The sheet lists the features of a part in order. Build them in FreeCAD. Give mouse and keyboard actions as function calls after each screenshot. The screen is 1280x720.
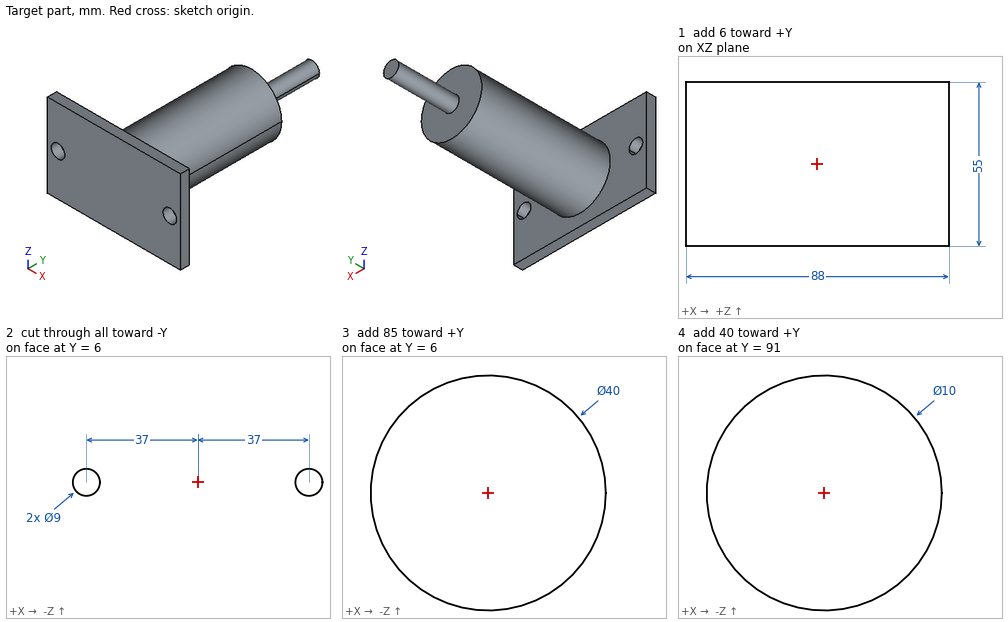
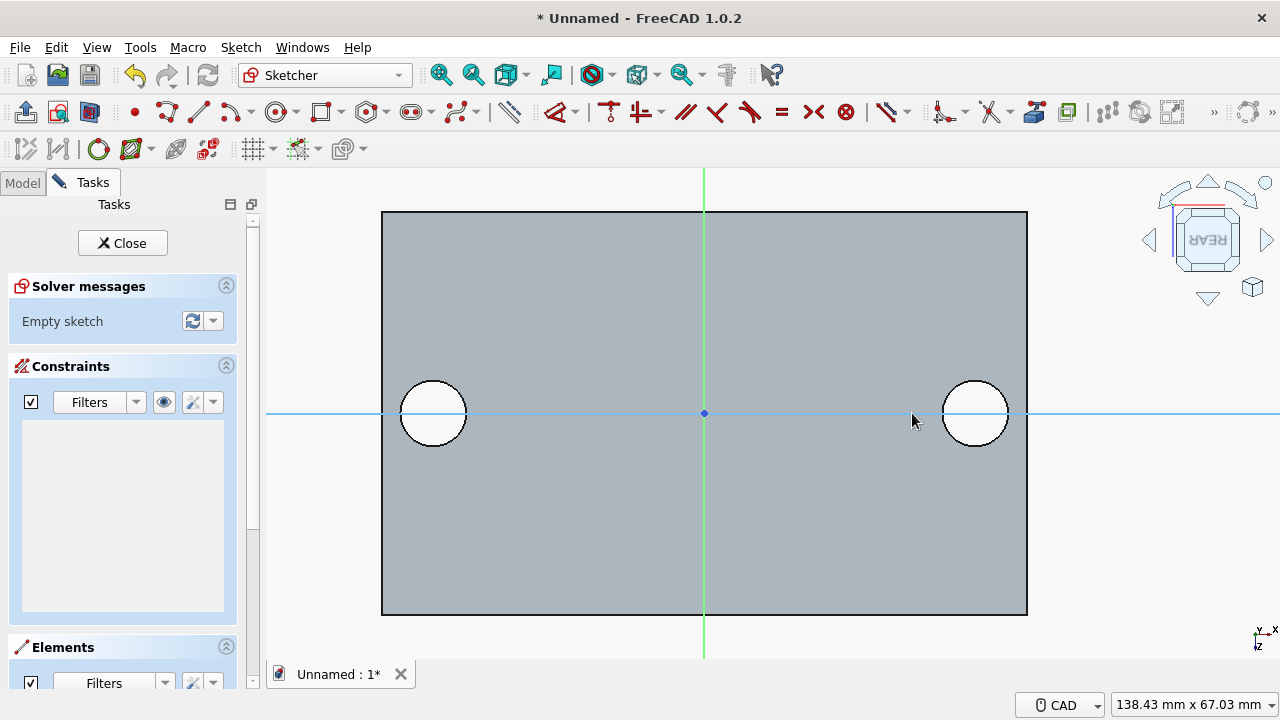
key(g)
key(c)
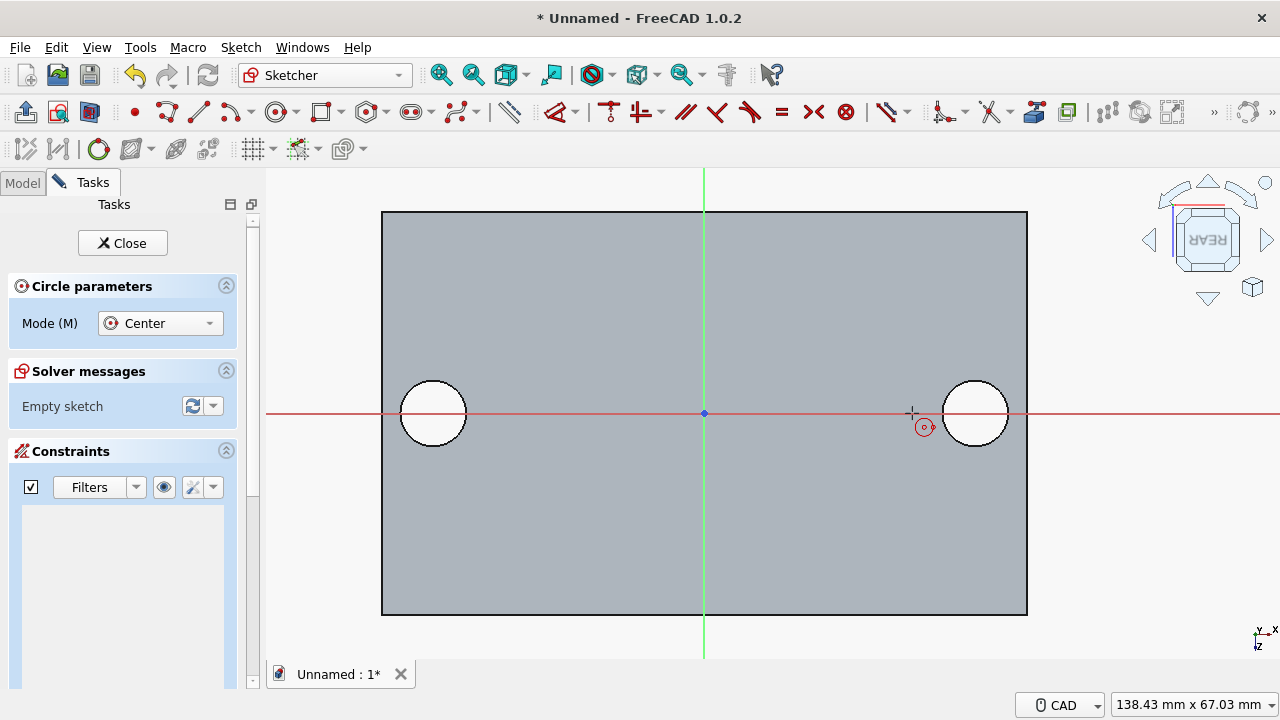
click(704, 413)
click(808, 310)
key(Escape)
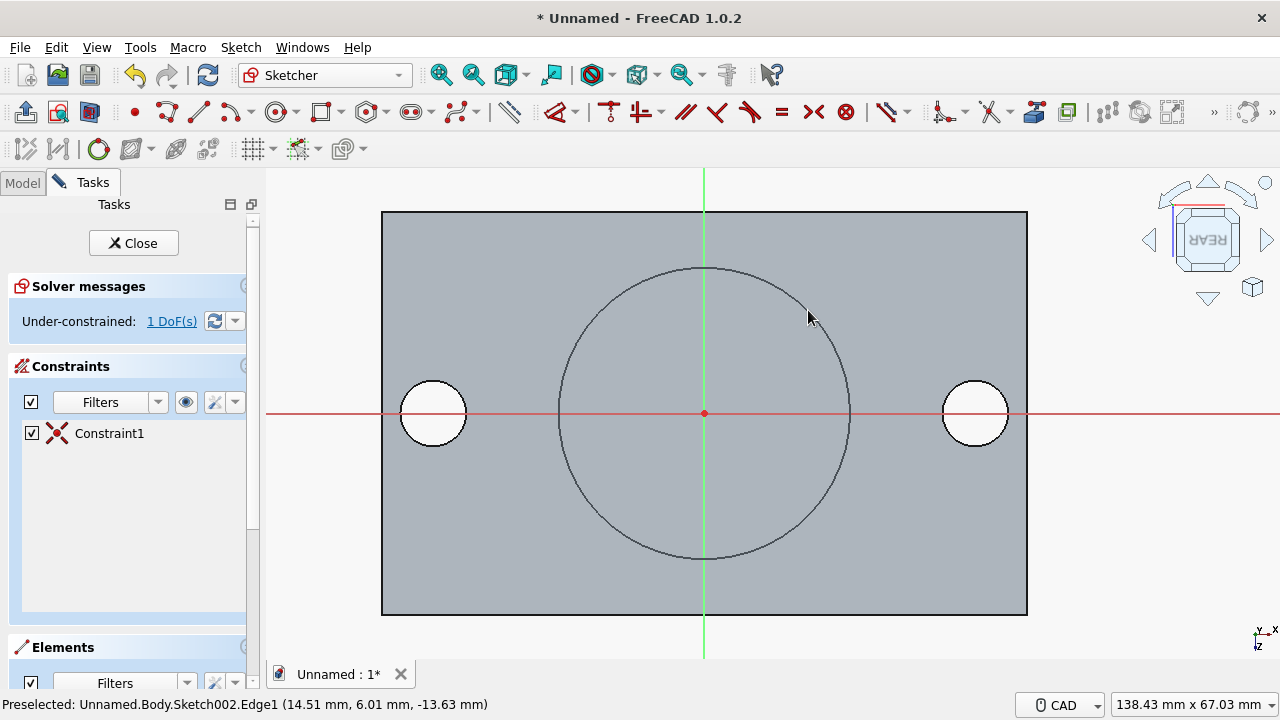
click(807, 310)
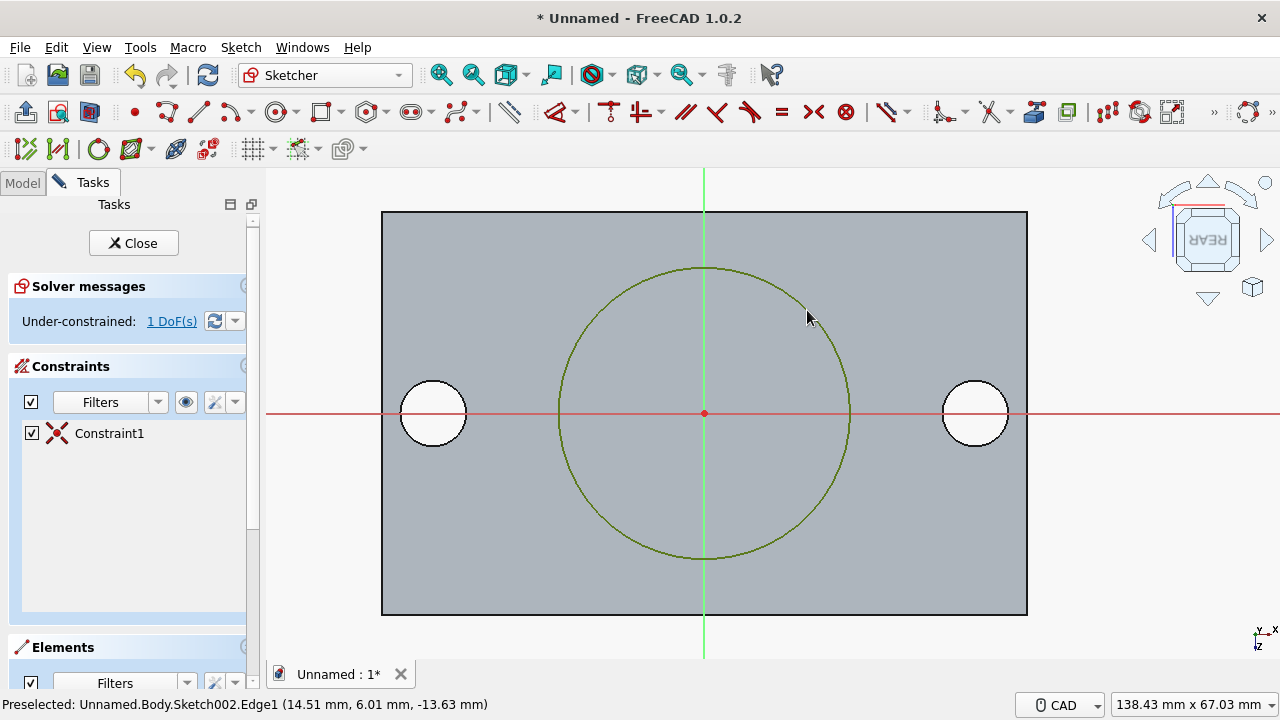
key(k)
key(o)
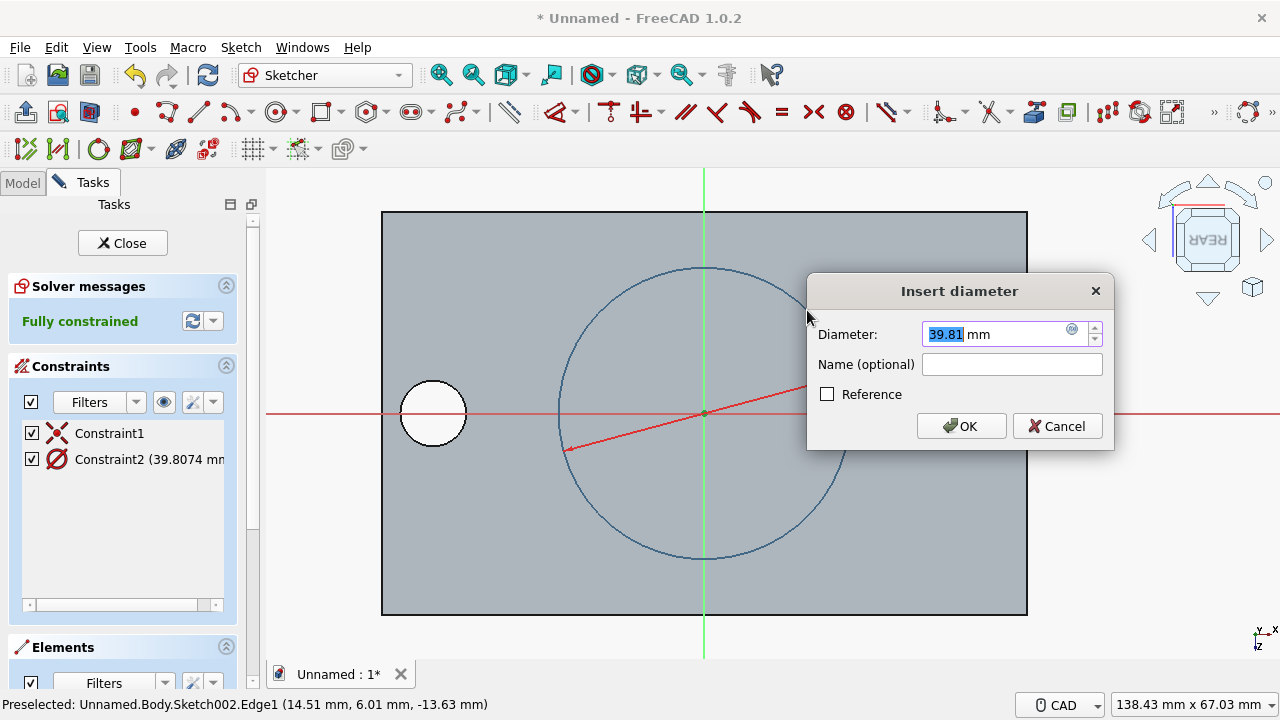
text(40)
key(Return)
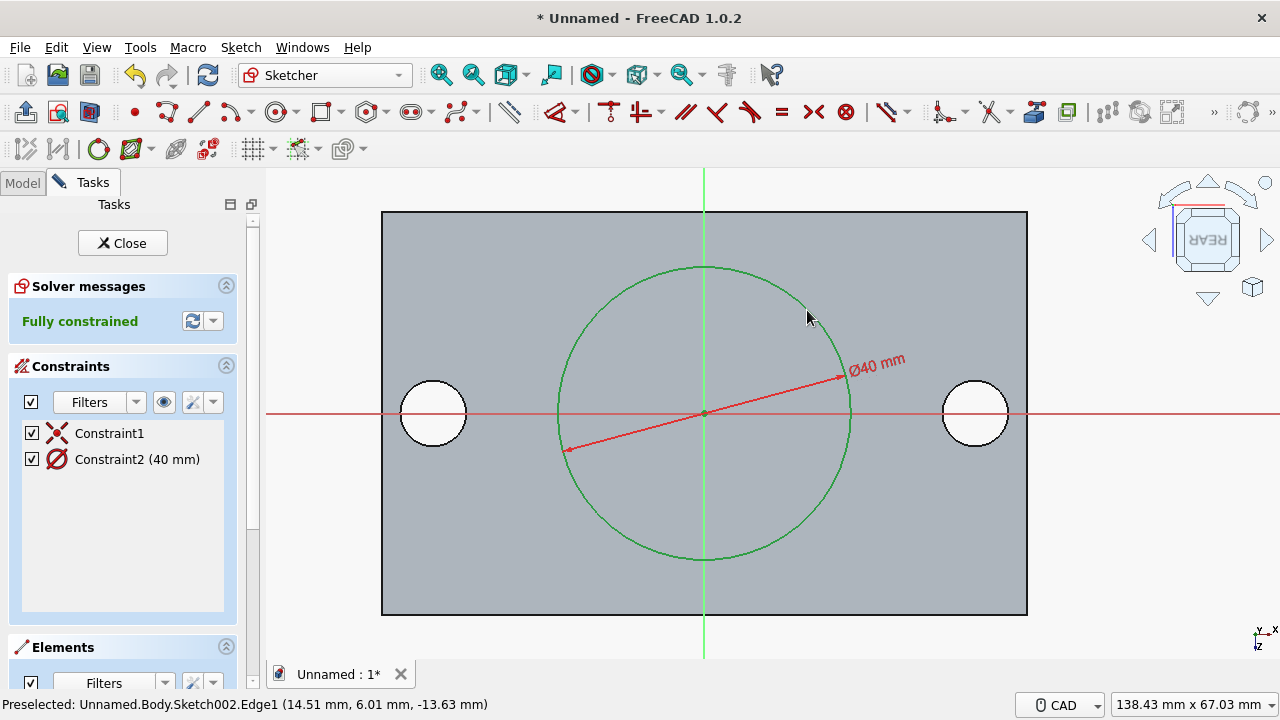
click(123, 243)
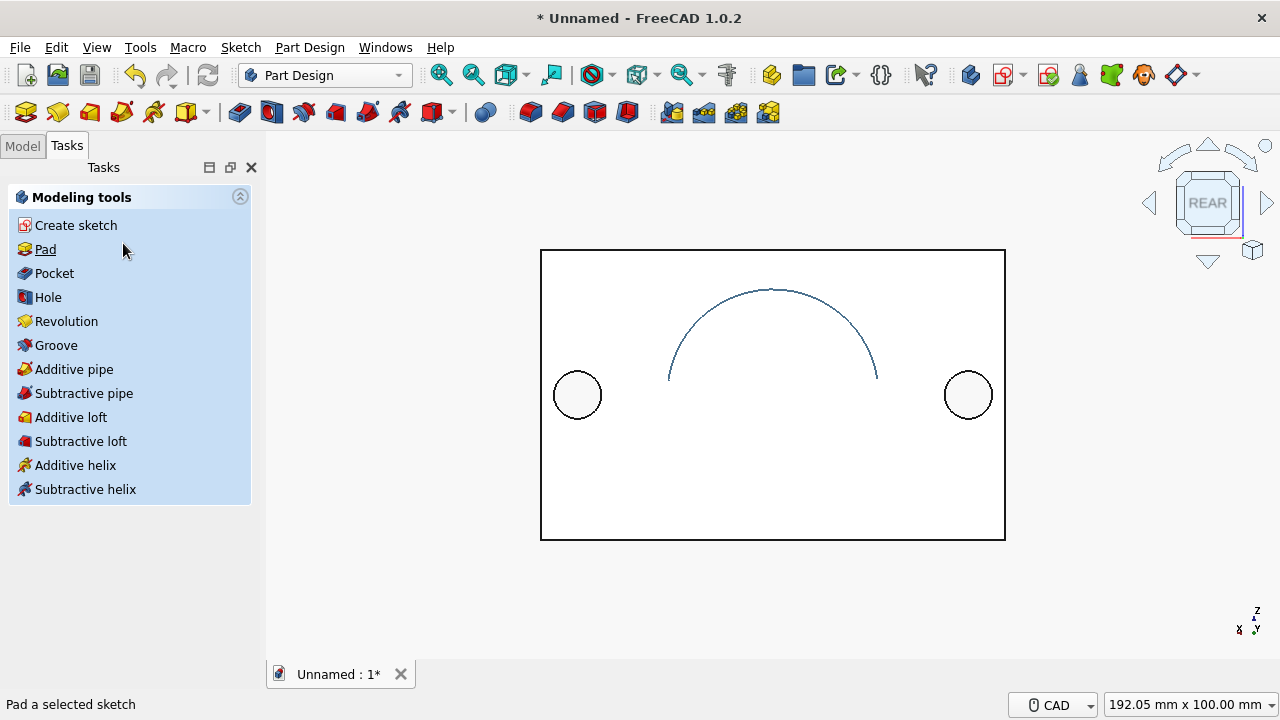
click(26, 112)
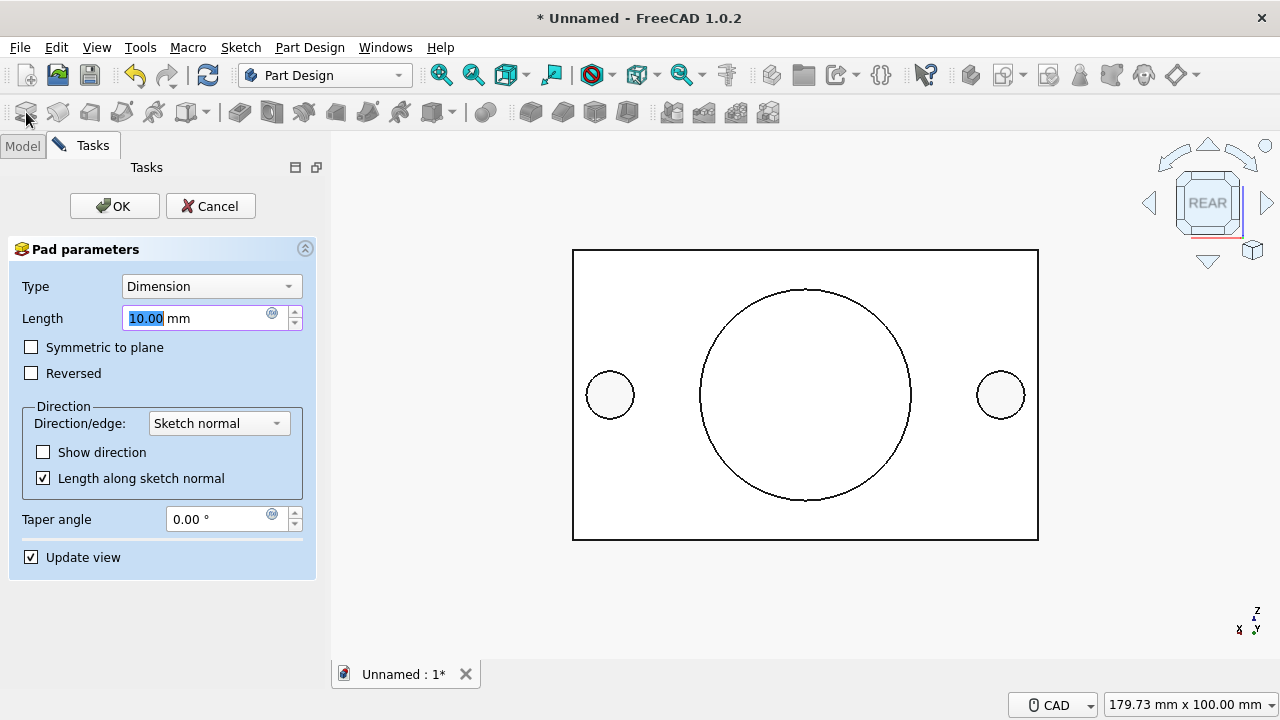
text(85)
key(Tab)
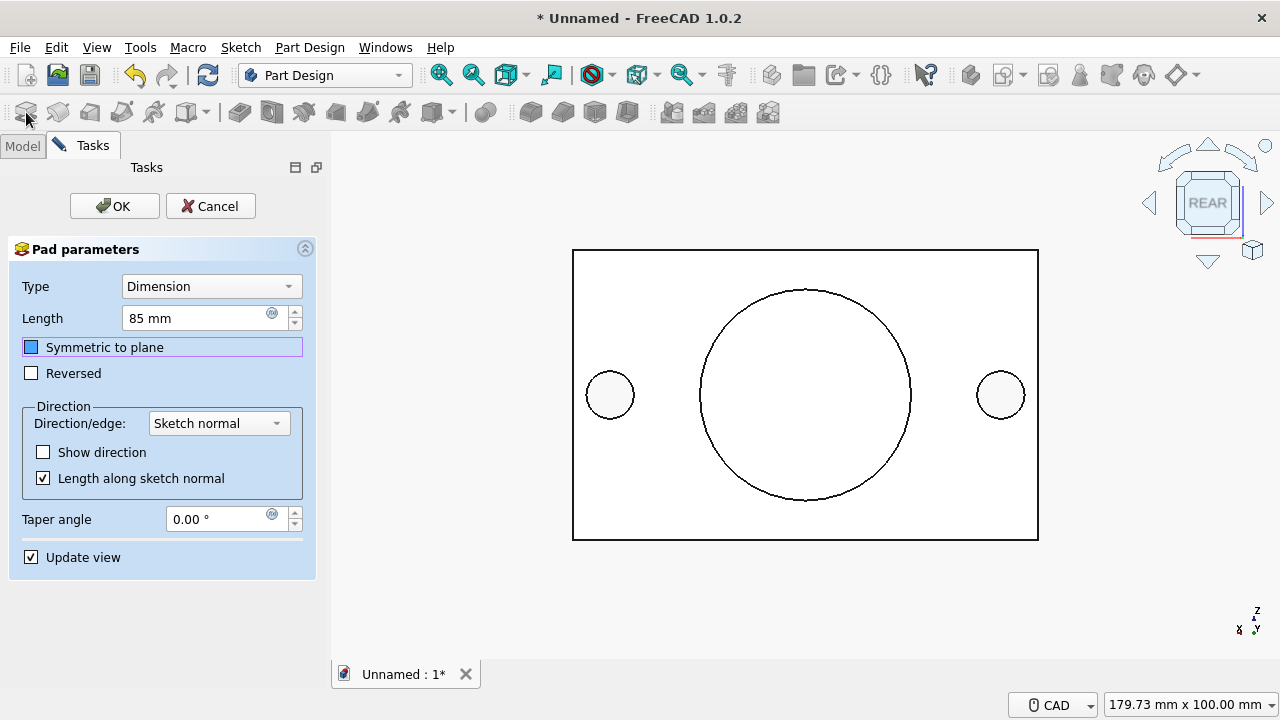
click(115, 206)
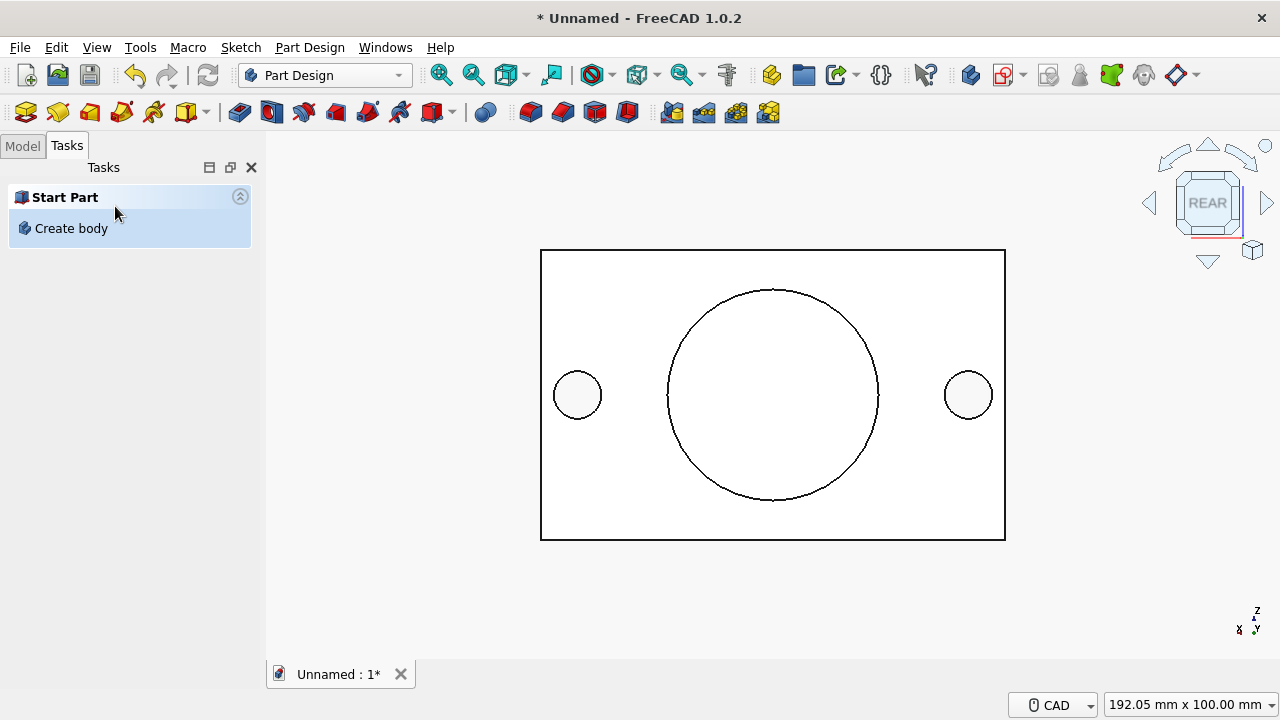
click(773, 394)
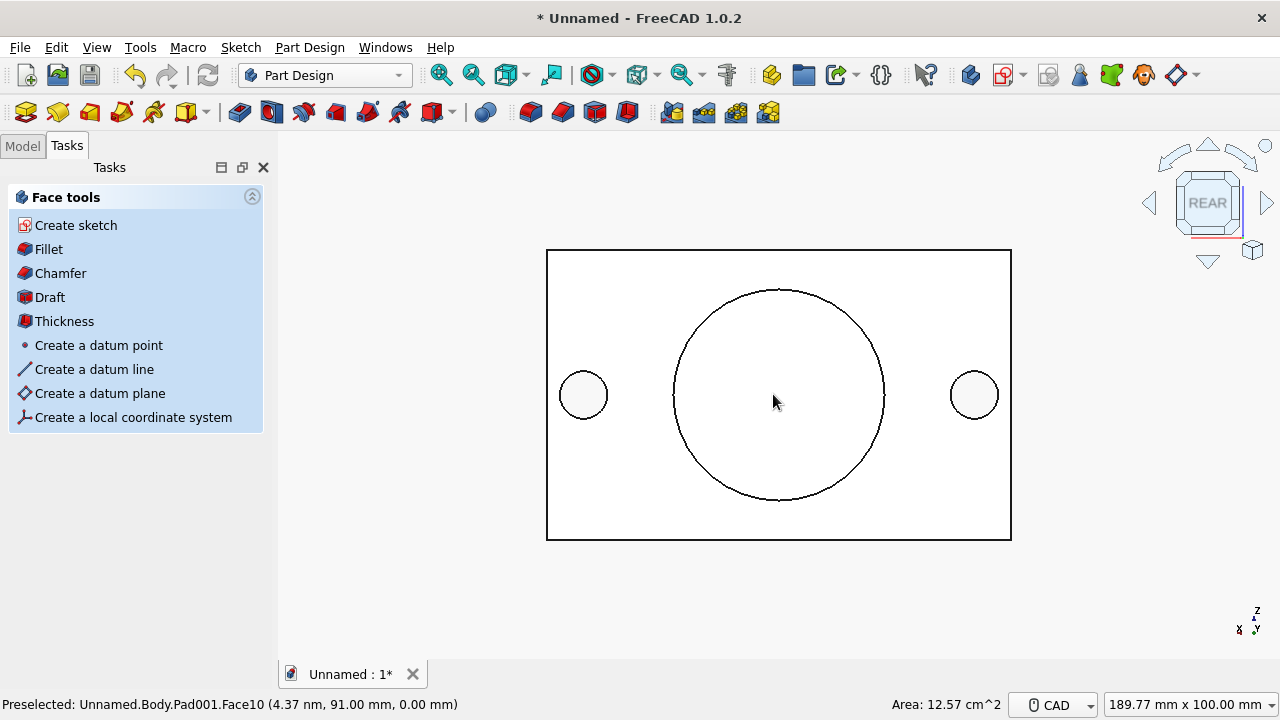
click(1004, 76)